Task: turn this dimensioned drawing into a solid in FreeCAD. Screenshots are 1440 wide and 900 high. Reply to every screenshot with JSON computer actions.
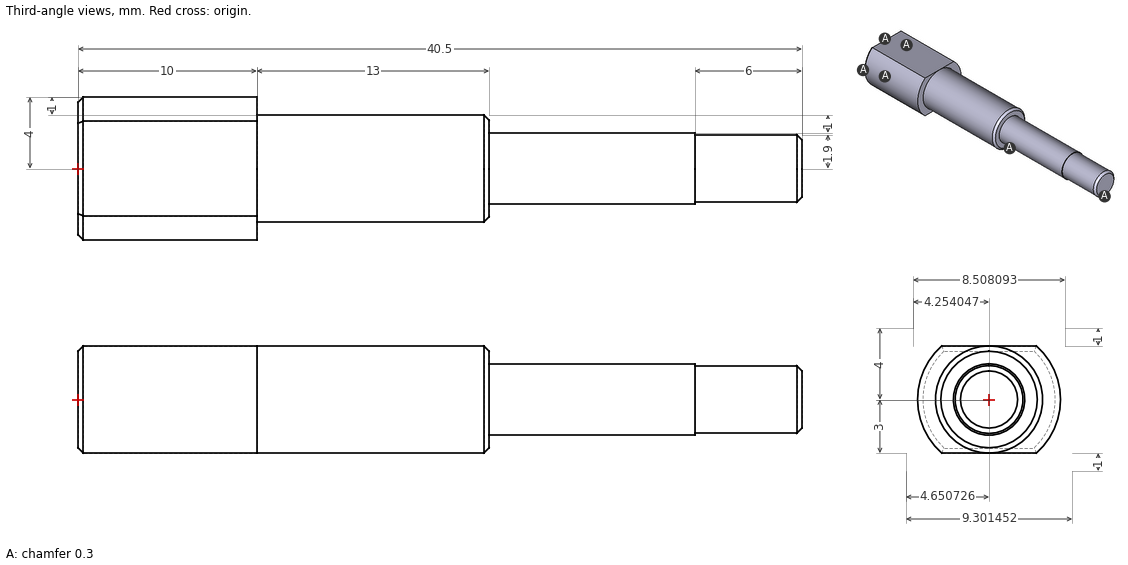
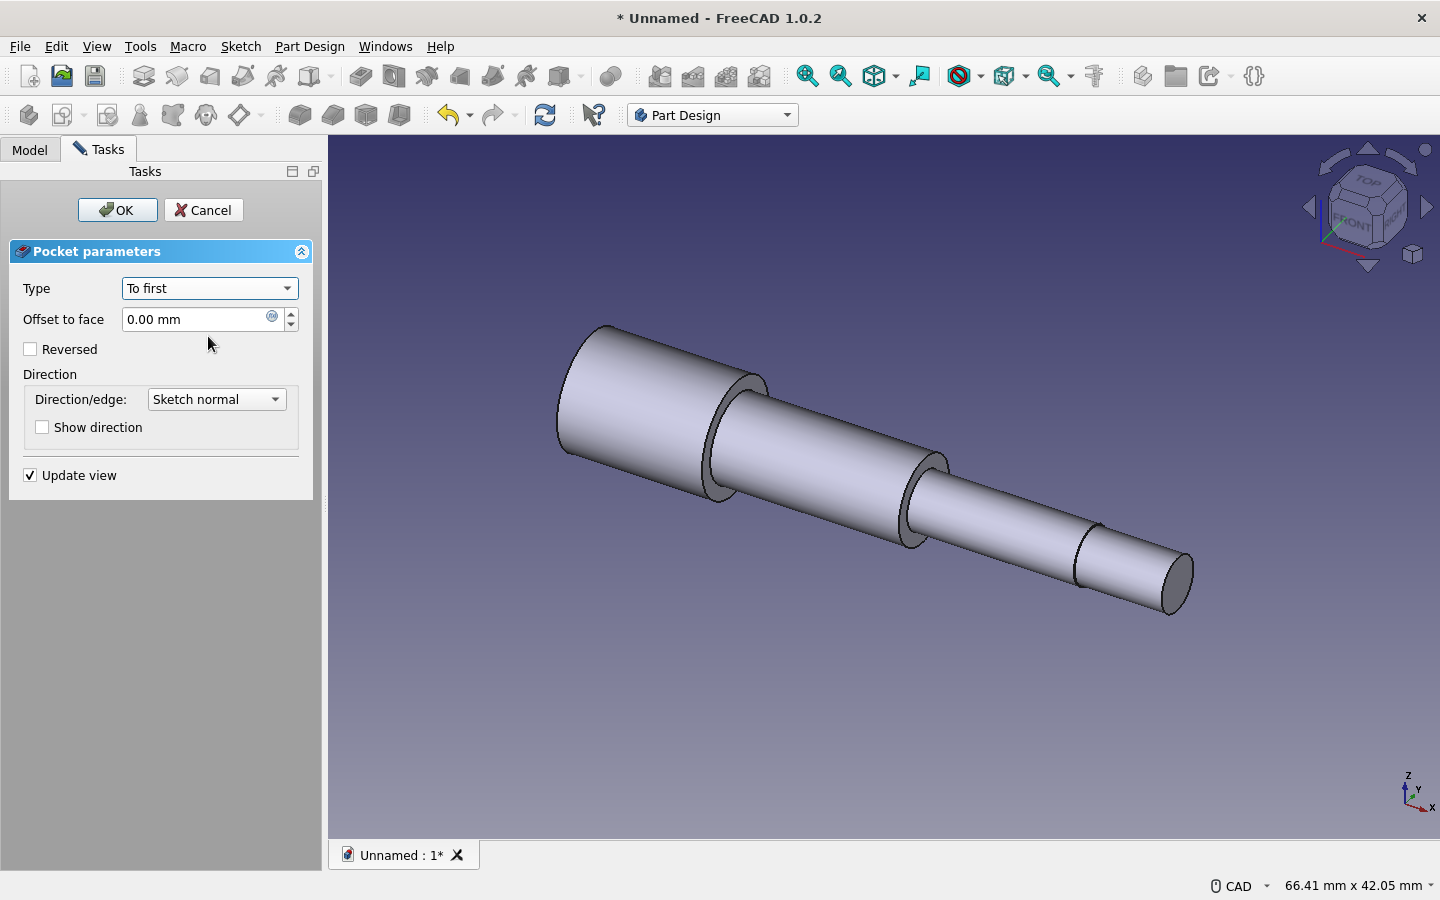
{"action": "left_click", "coordinate": [31, 349]}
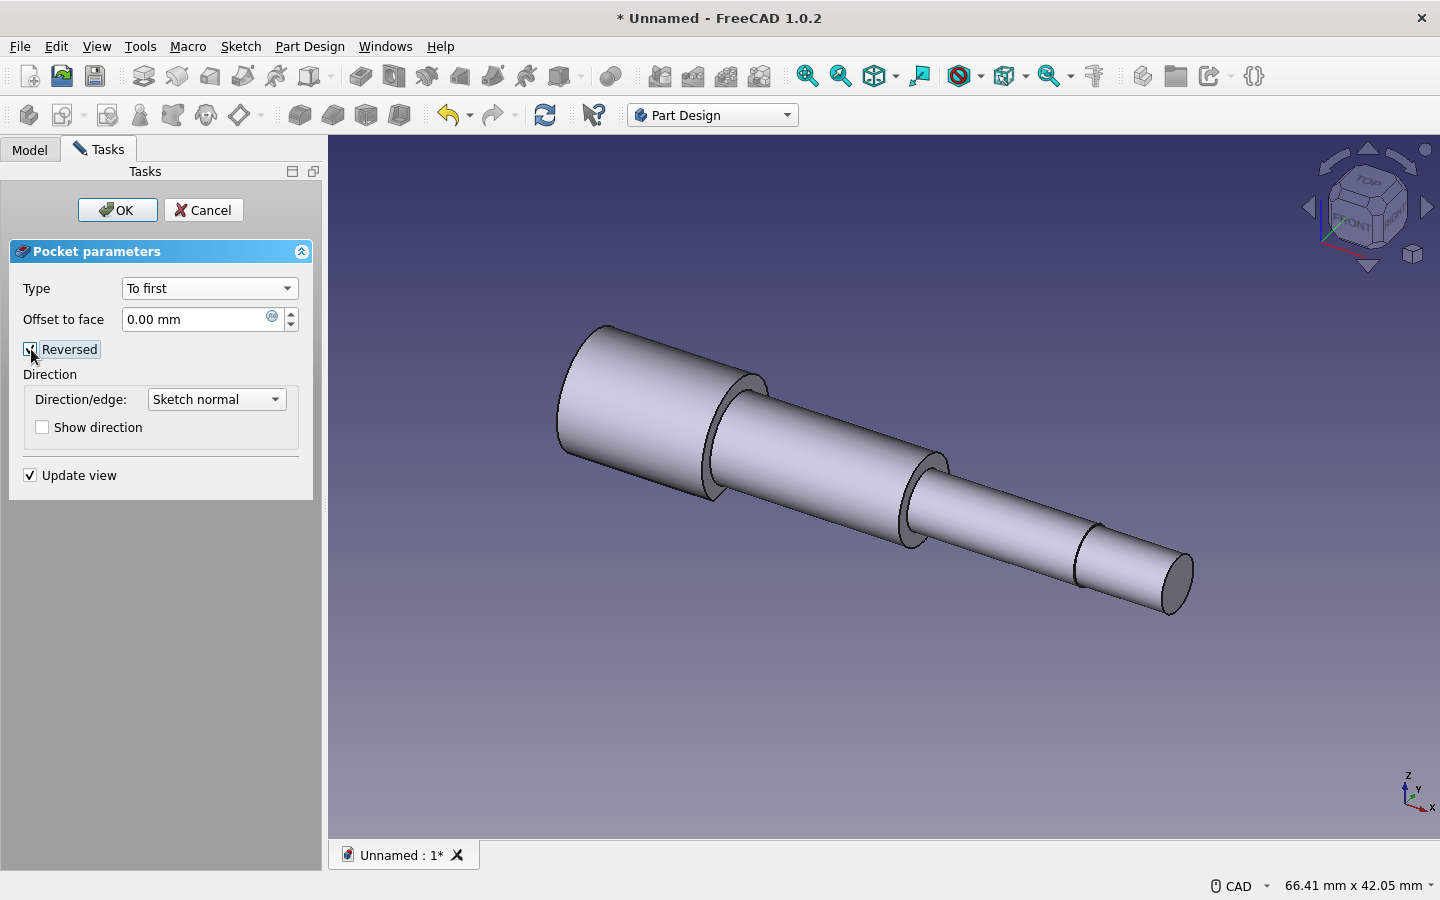
{"action": "left_click", "coordinate": [118, 210]}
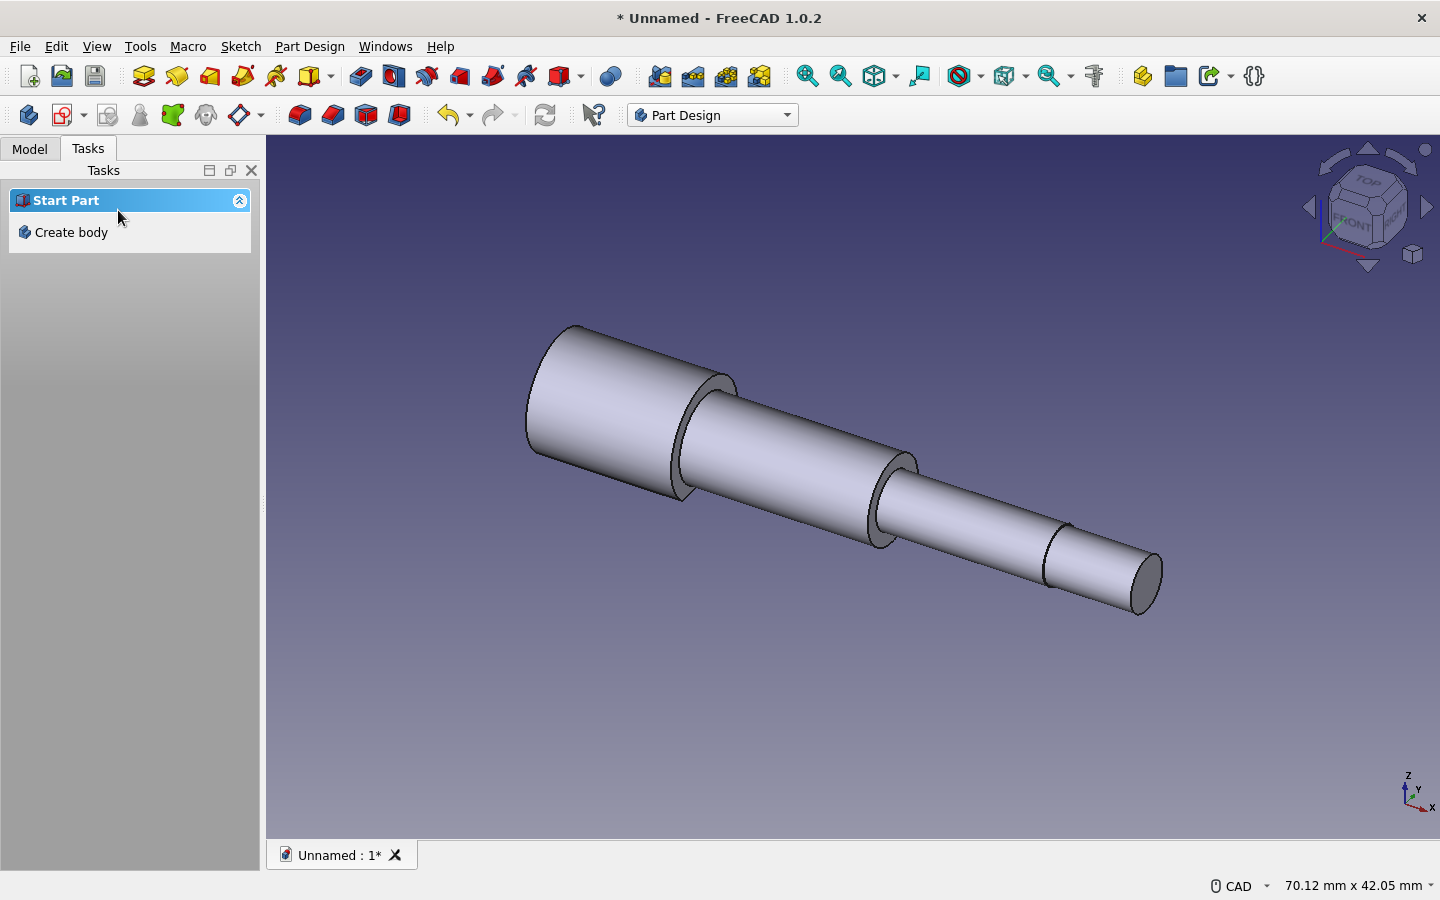
{"action": "left_click", "coordinate": [62, 116]}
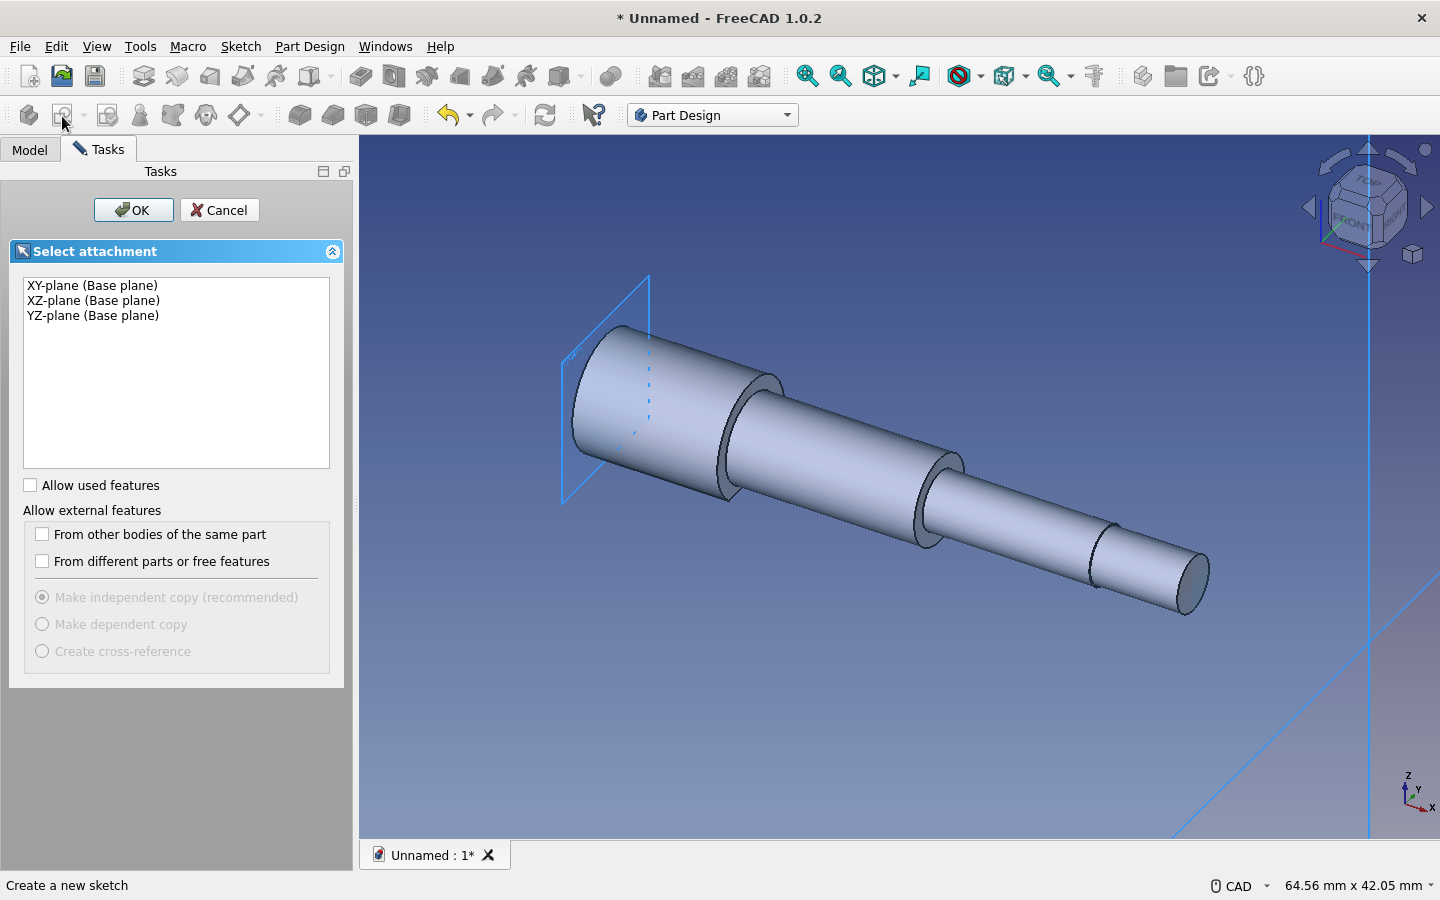
{"action": "left_click", "coordinate": [84, 316]}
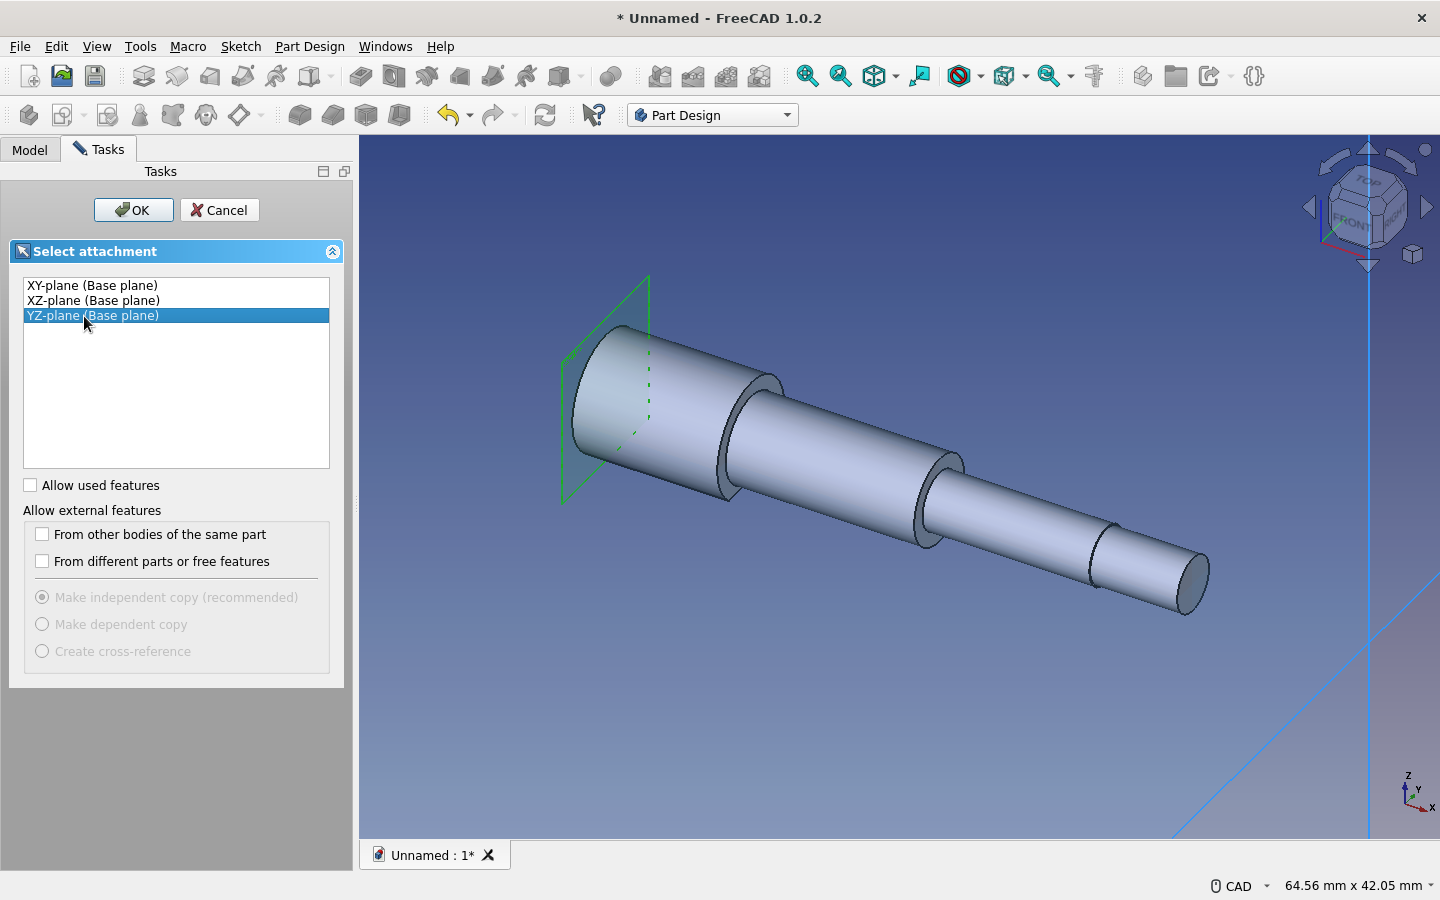
{"action": "left_click", "coordinate": [134, 210]}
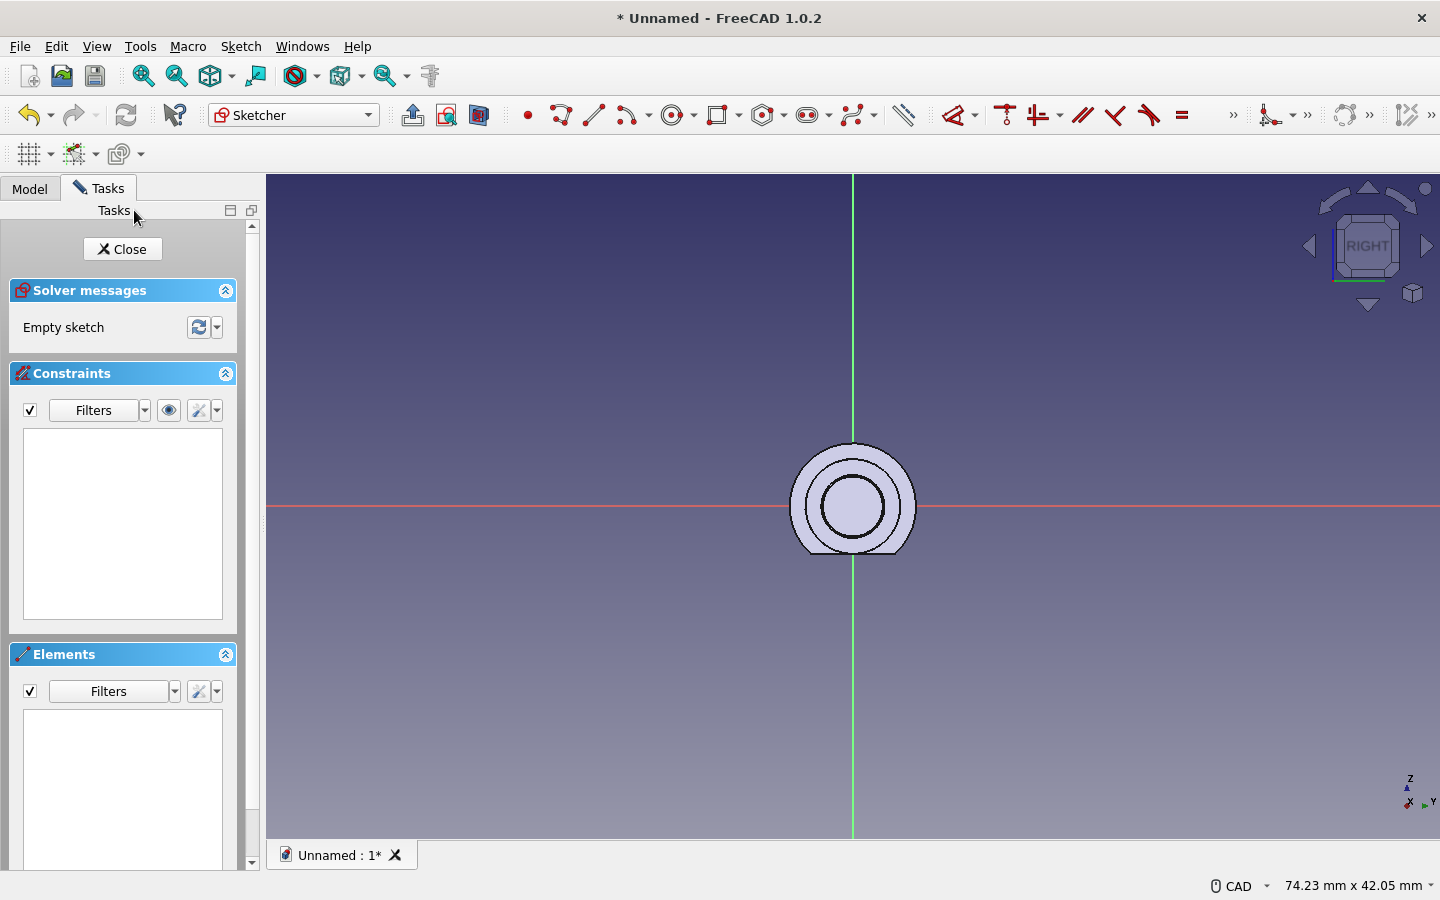
{"action": "key", "text": "q s"}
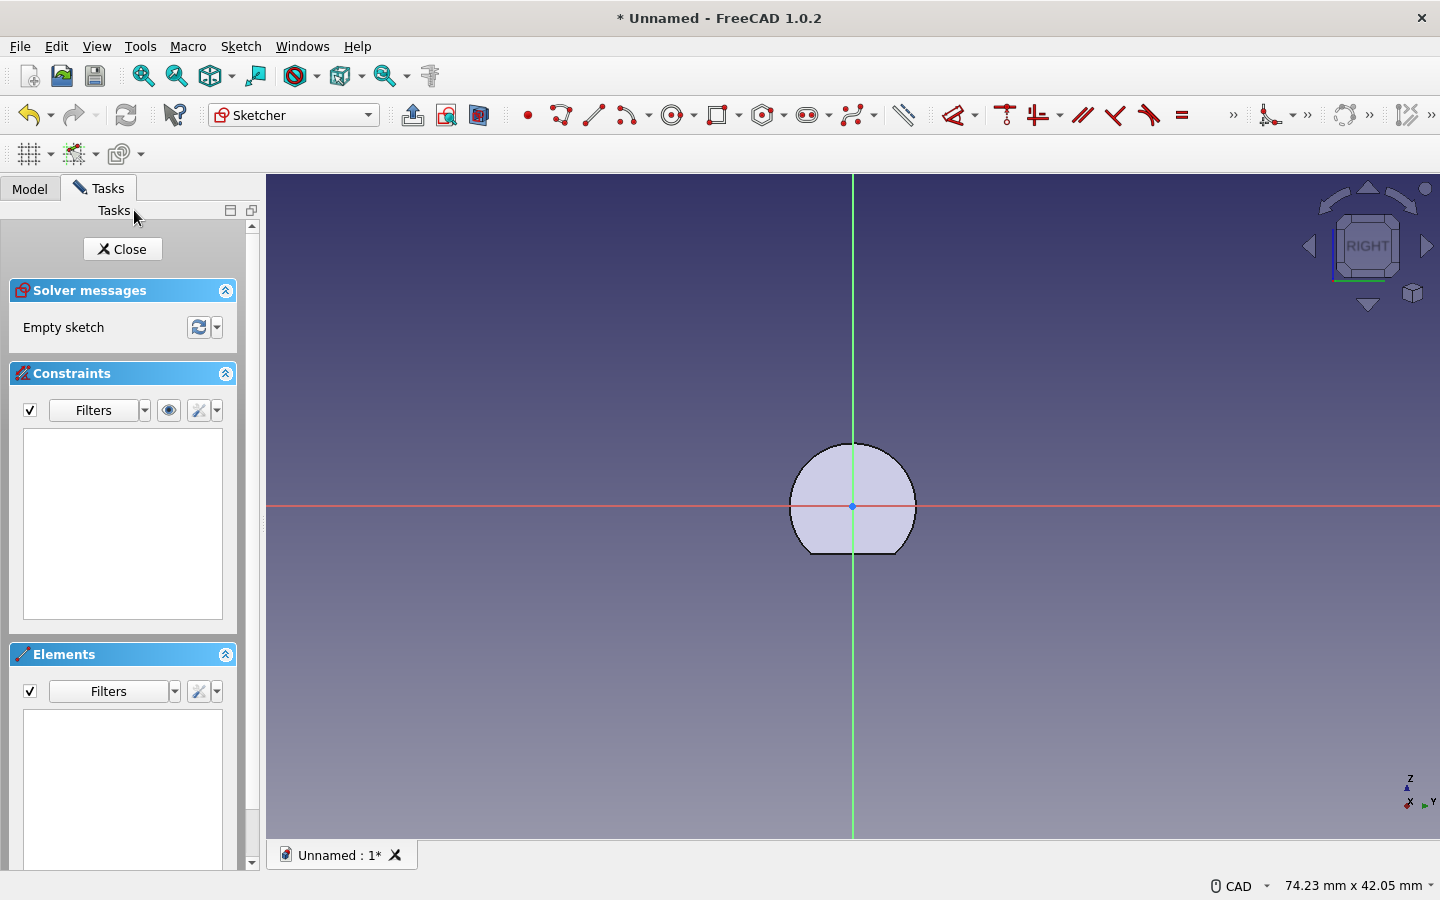
{"action": "scroll", "coordinate": [870, 467], "scroll_direction": "up", "scroll_amount": 8}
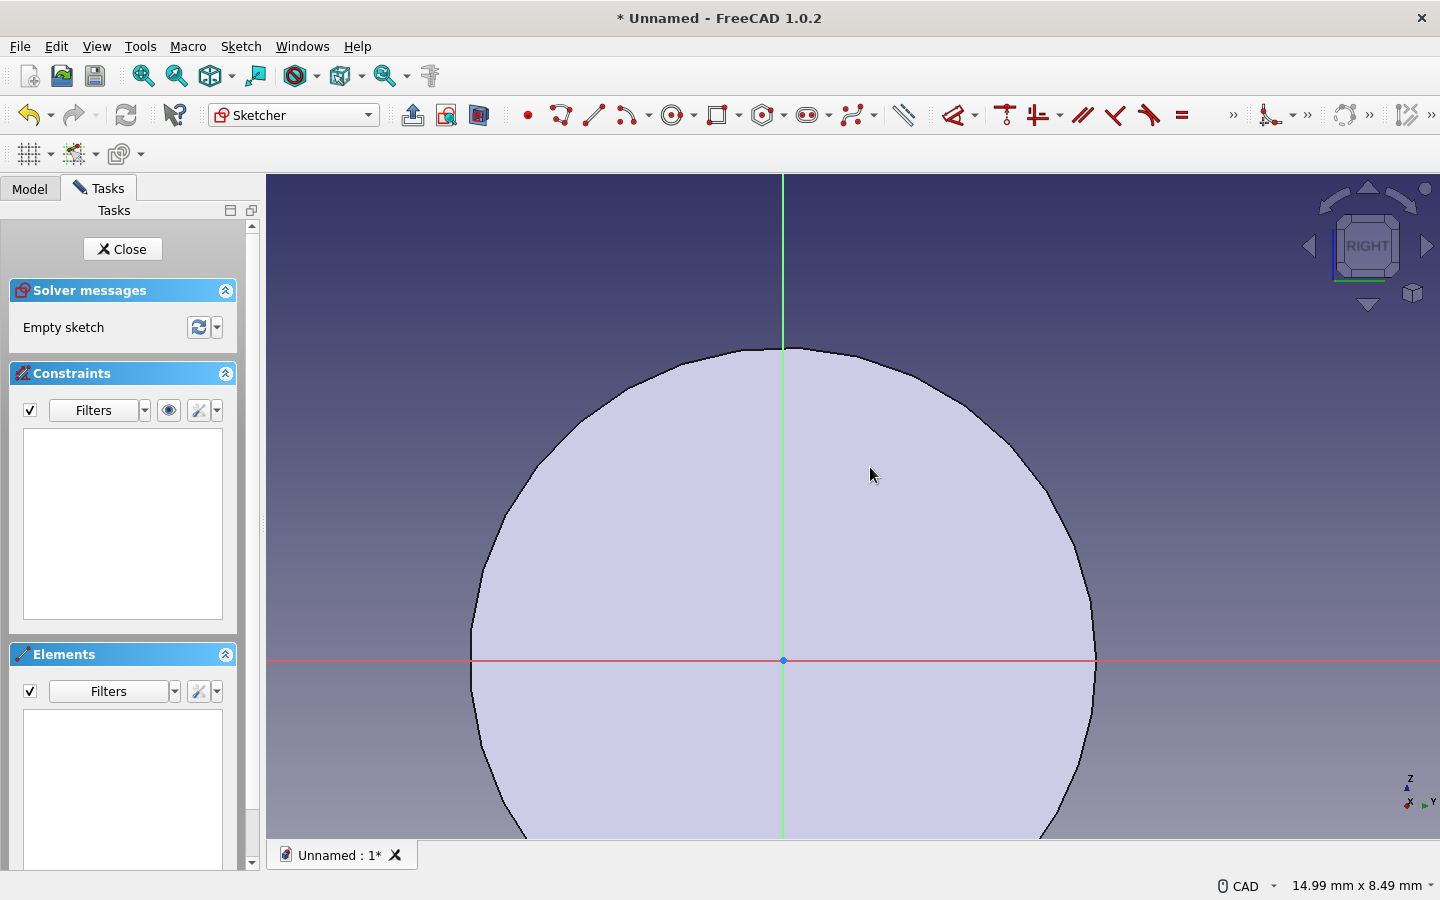
{"action": "key", "text": "g r"}